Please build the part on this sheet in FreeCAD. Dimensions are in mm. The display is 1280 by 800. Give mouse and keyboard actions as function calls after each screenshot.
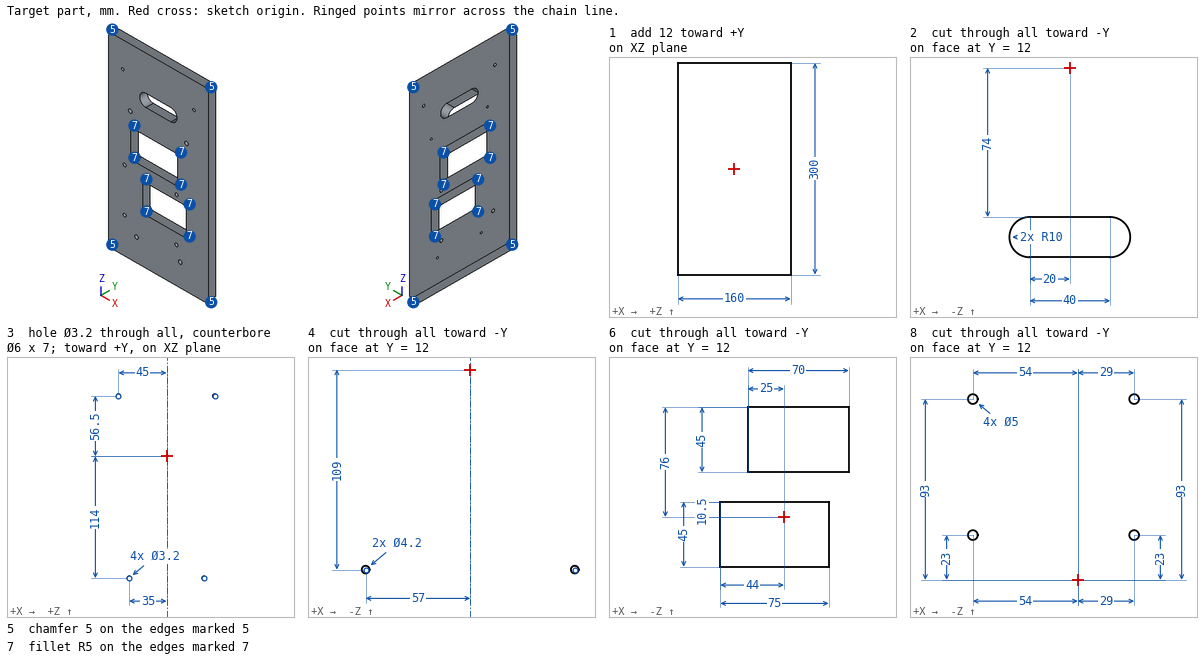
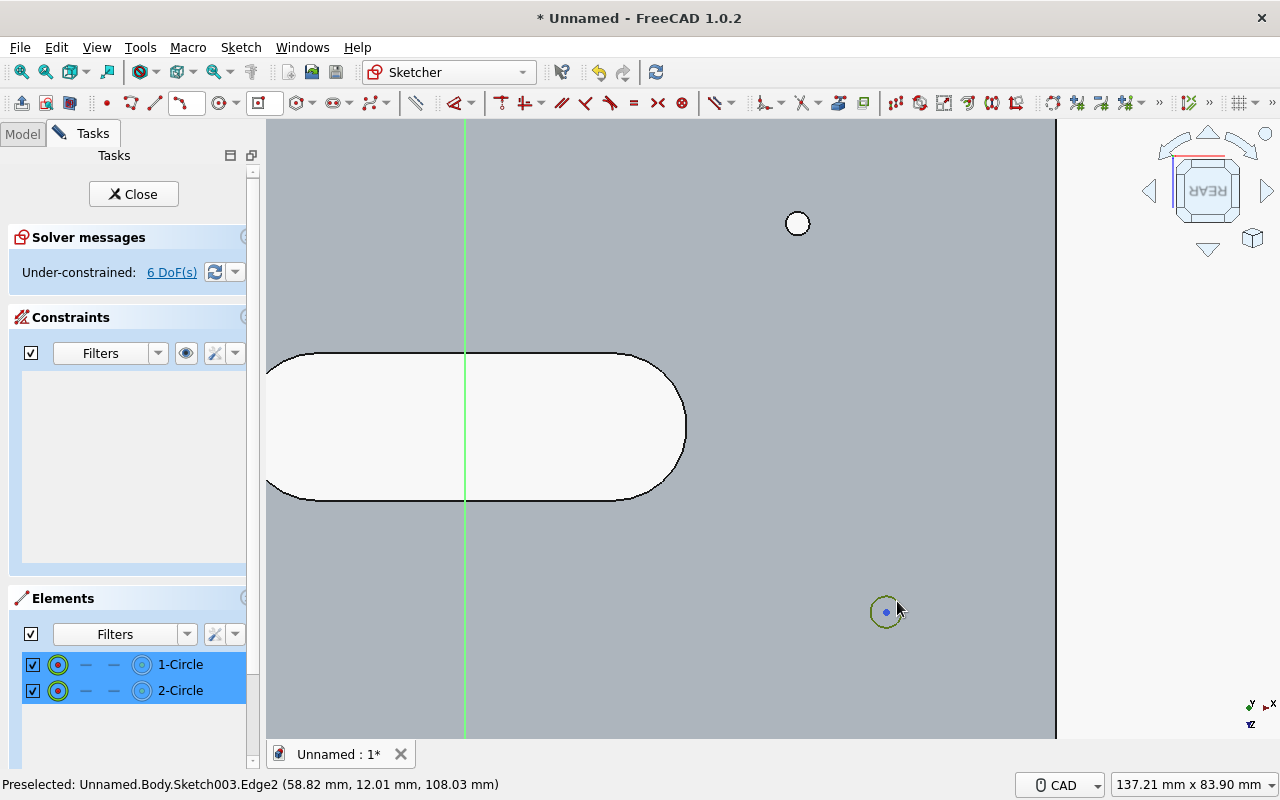
click(634, 104)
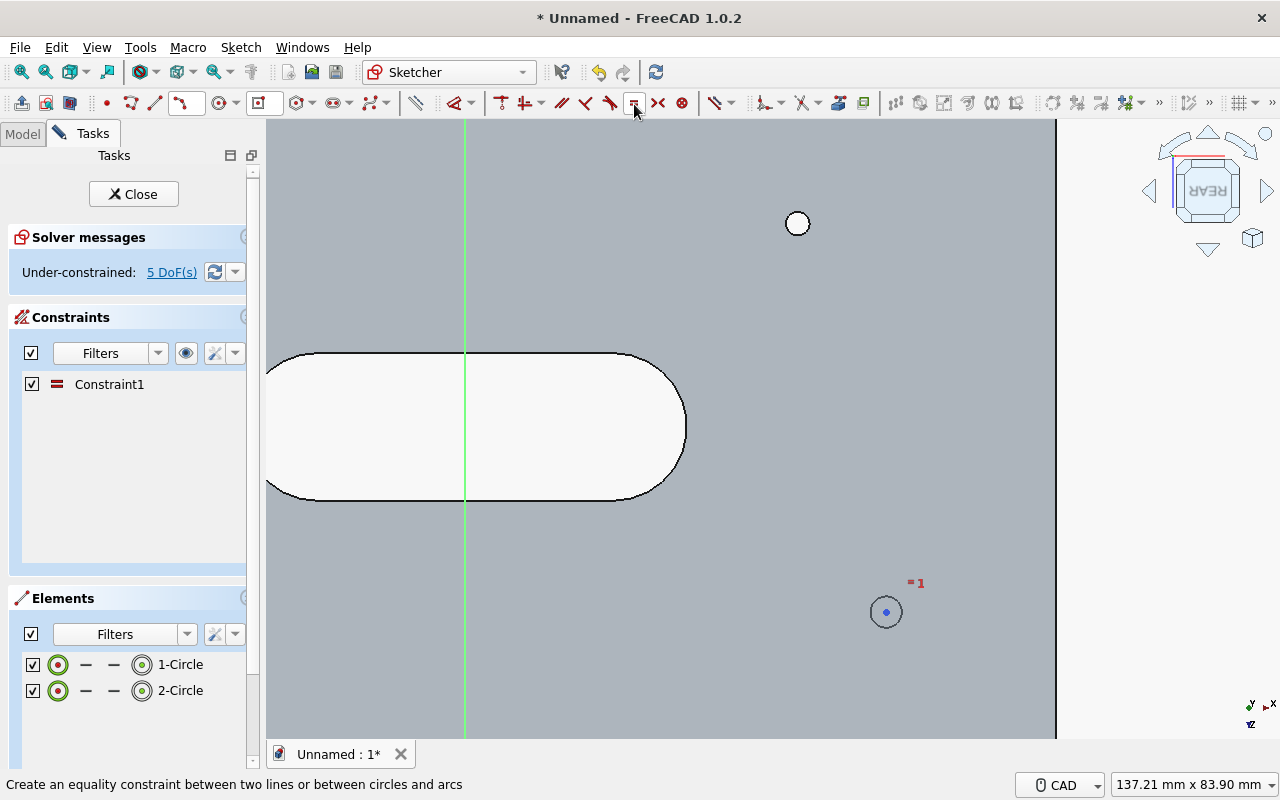
scroll(900, 602, down, 4)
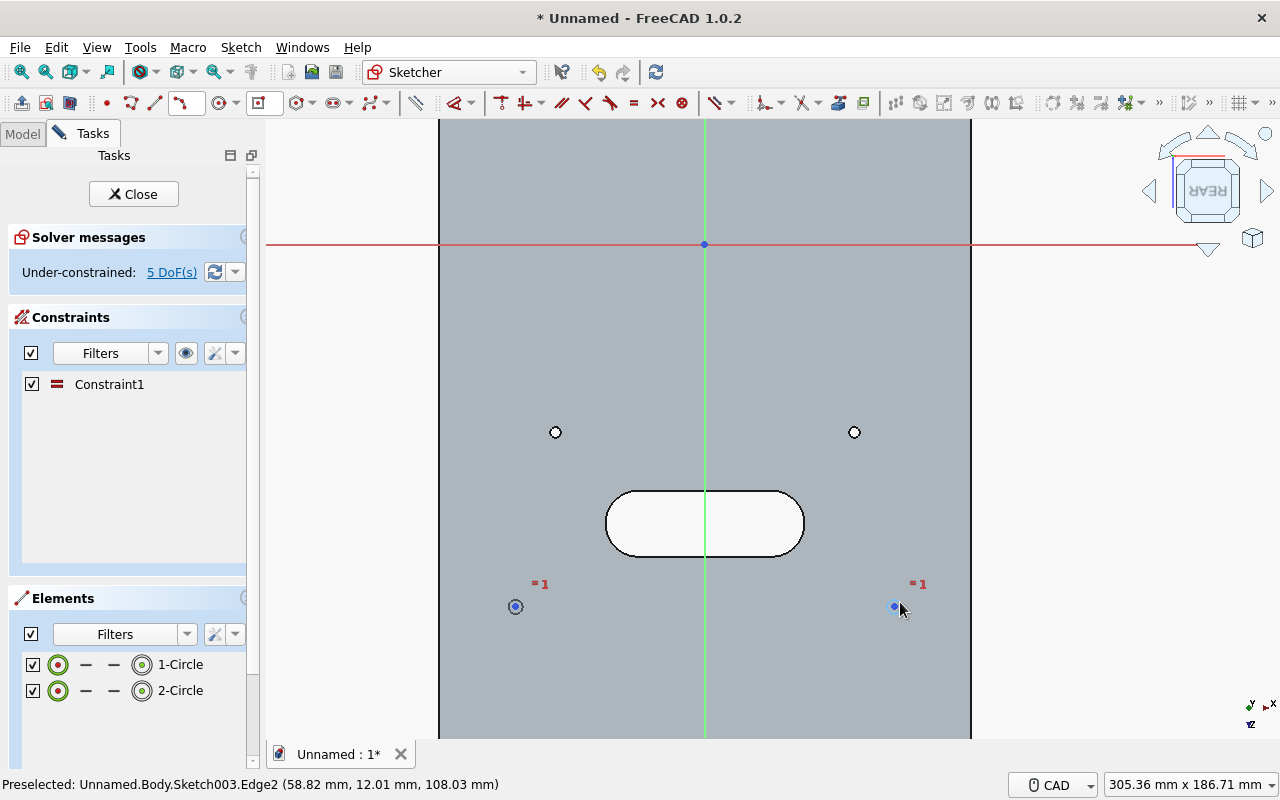
click(516, 607)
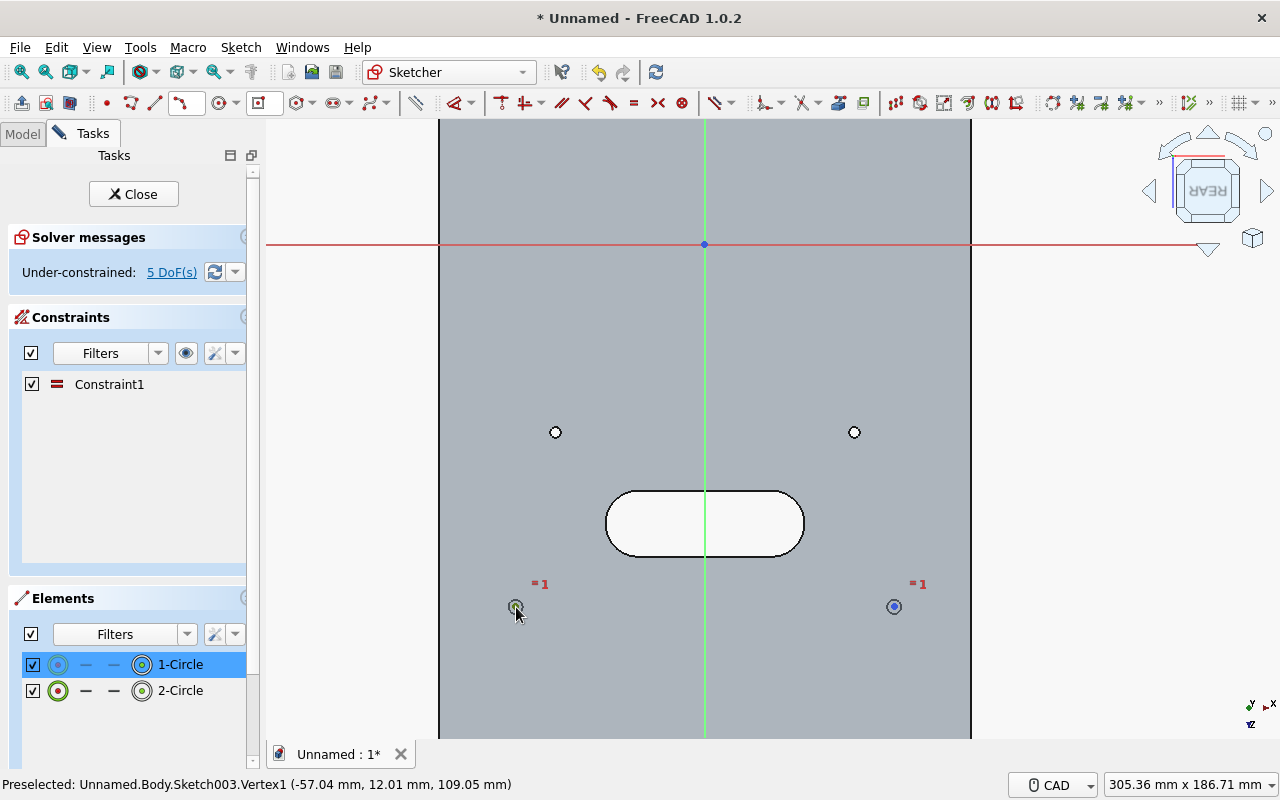
click(894, 607)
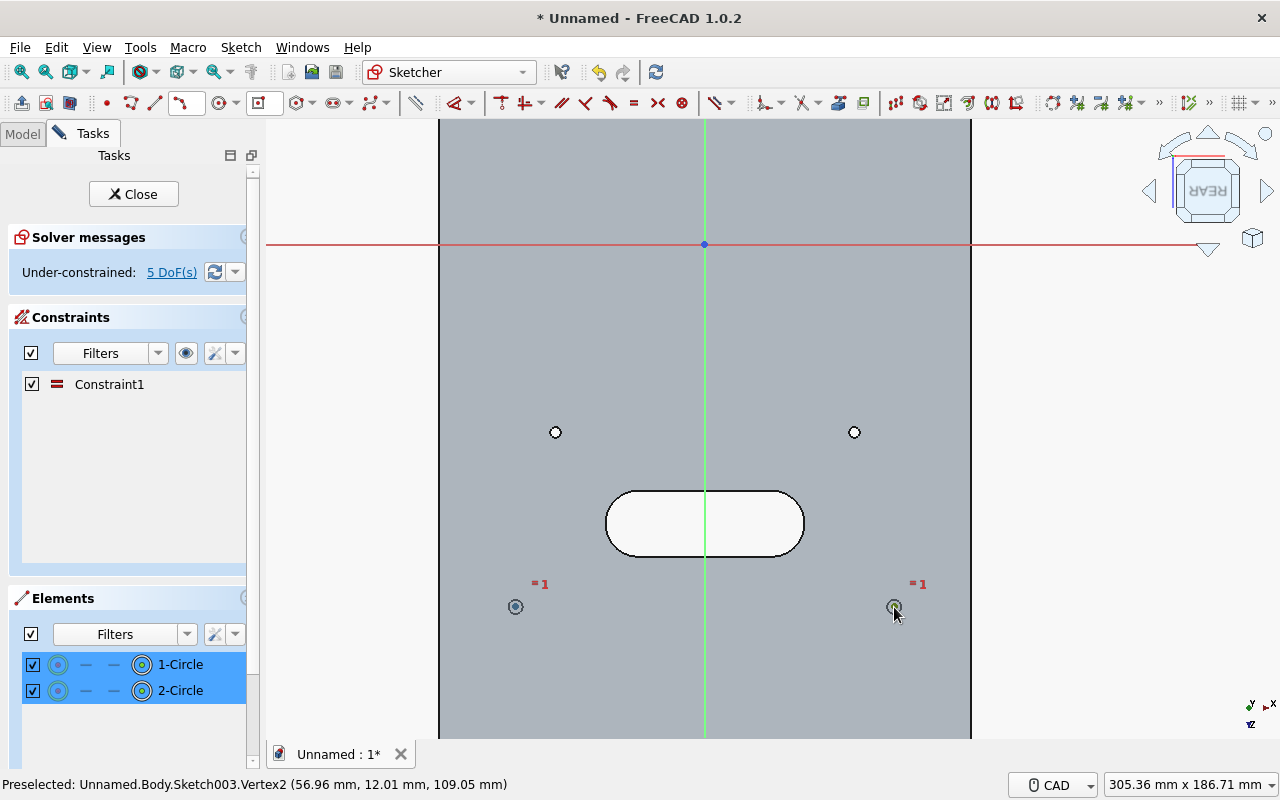
click(705, 671)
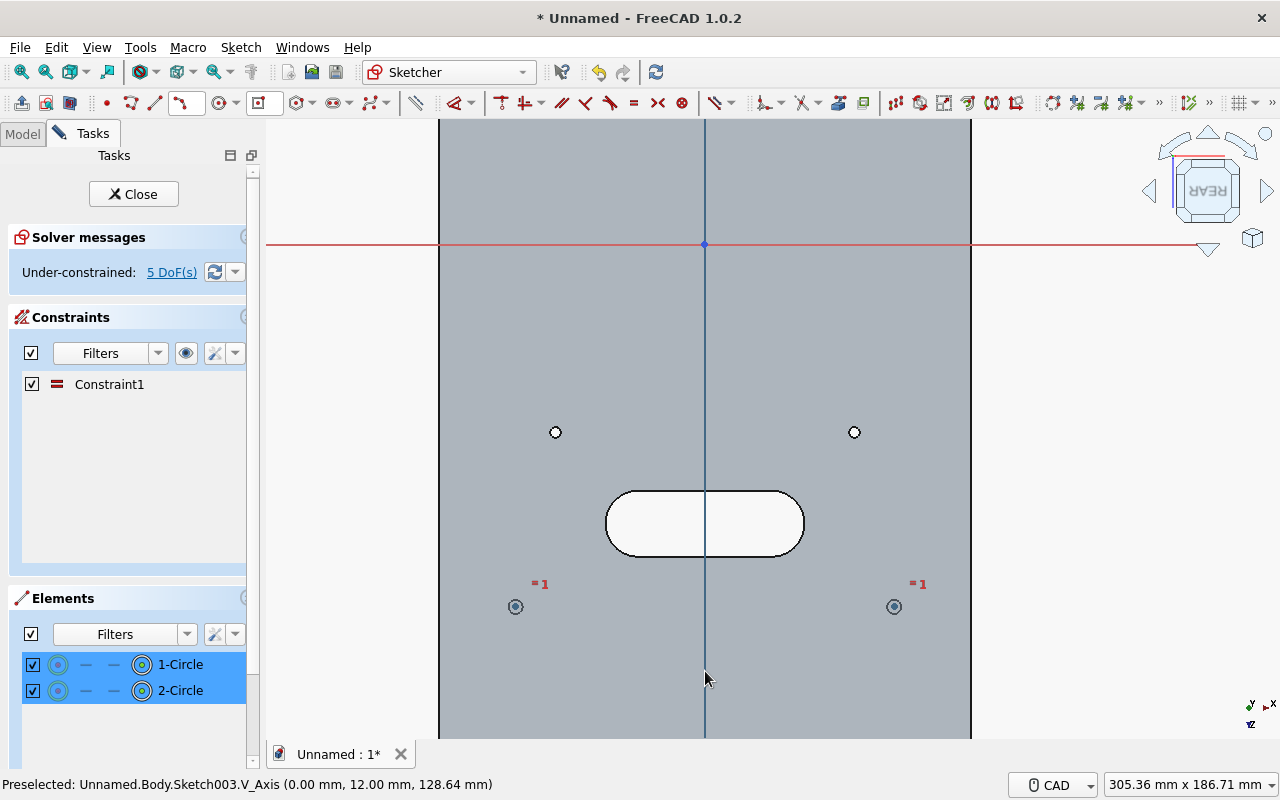
click(658, 104)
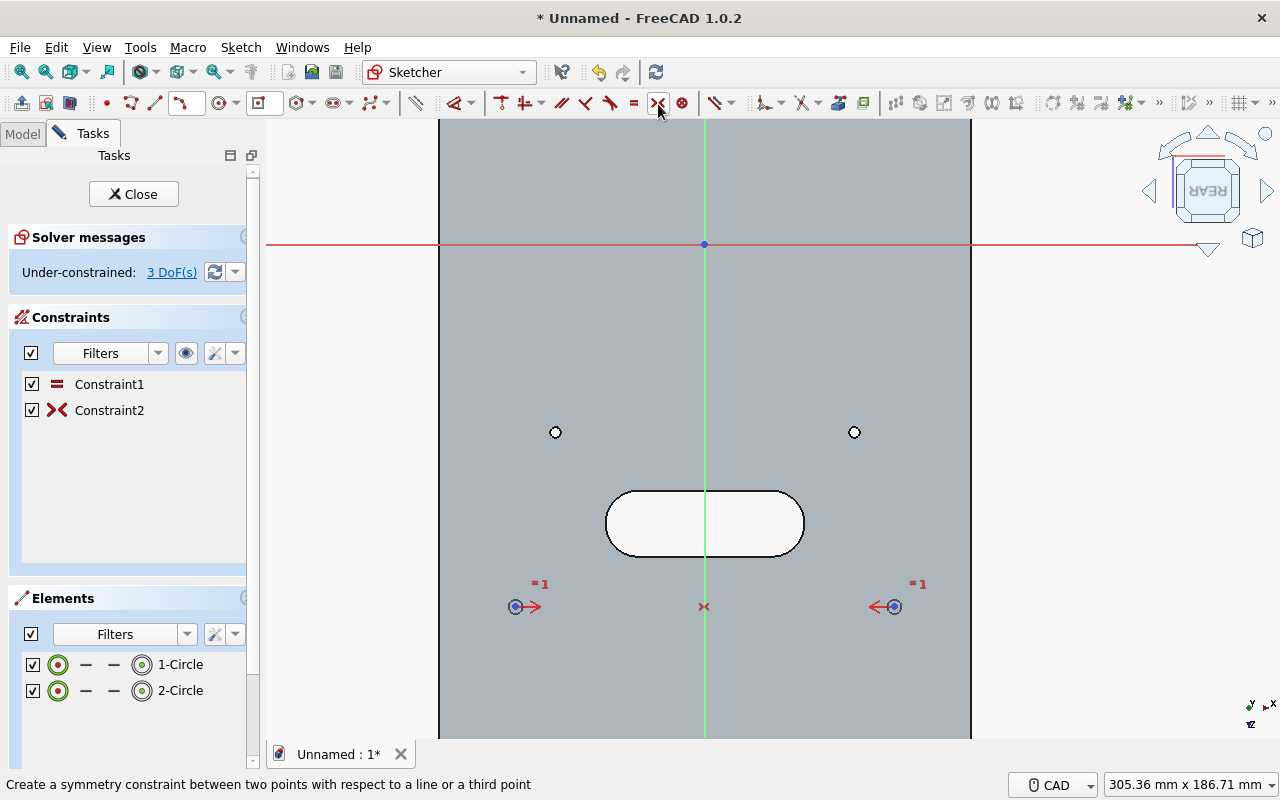
click(454, 104)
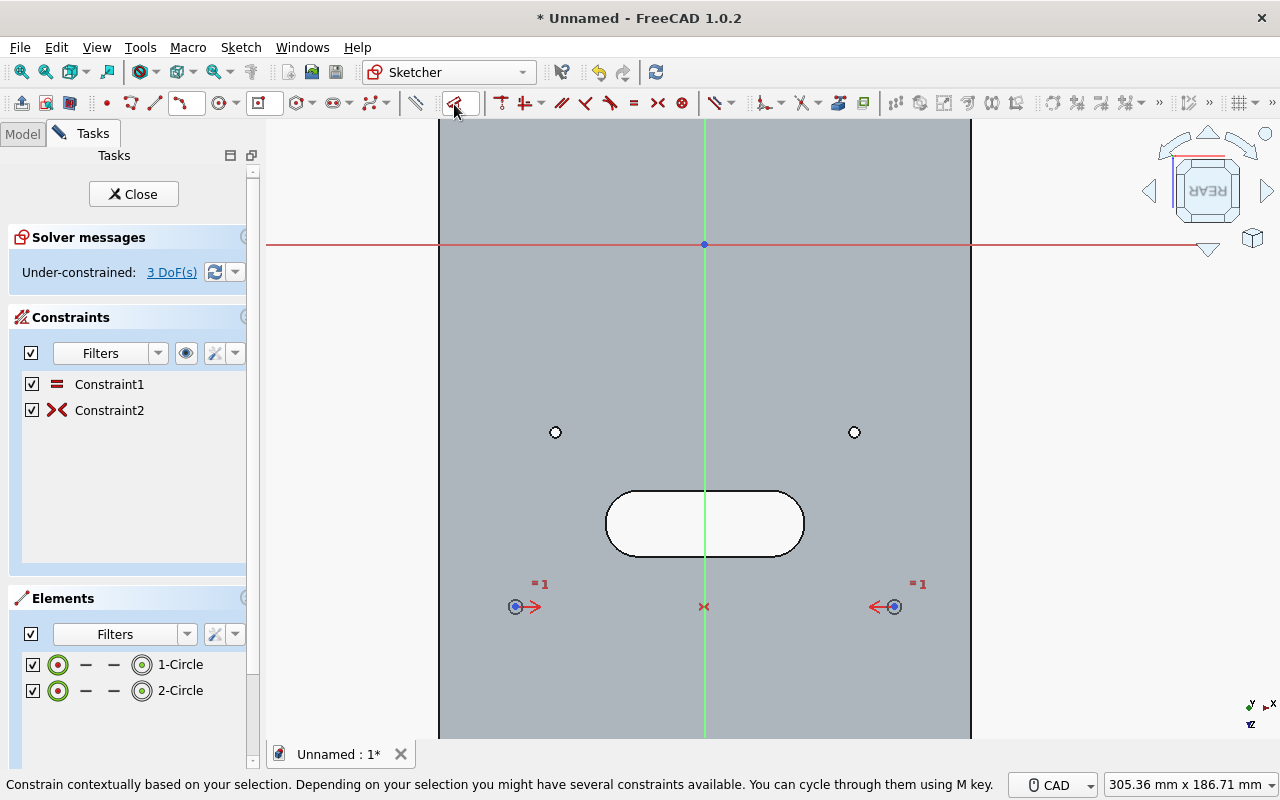
scroll(516, 600, up, 6)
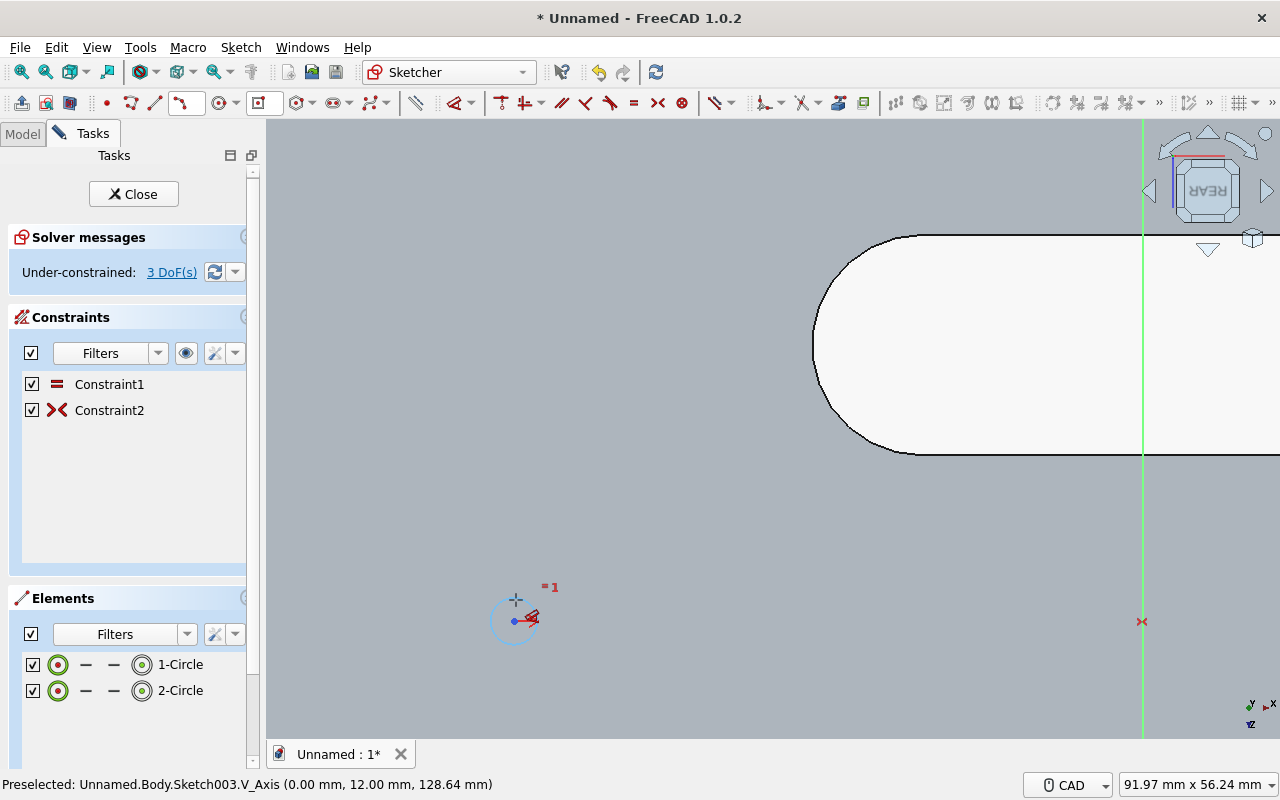
click(515, 598)
click(516, 566)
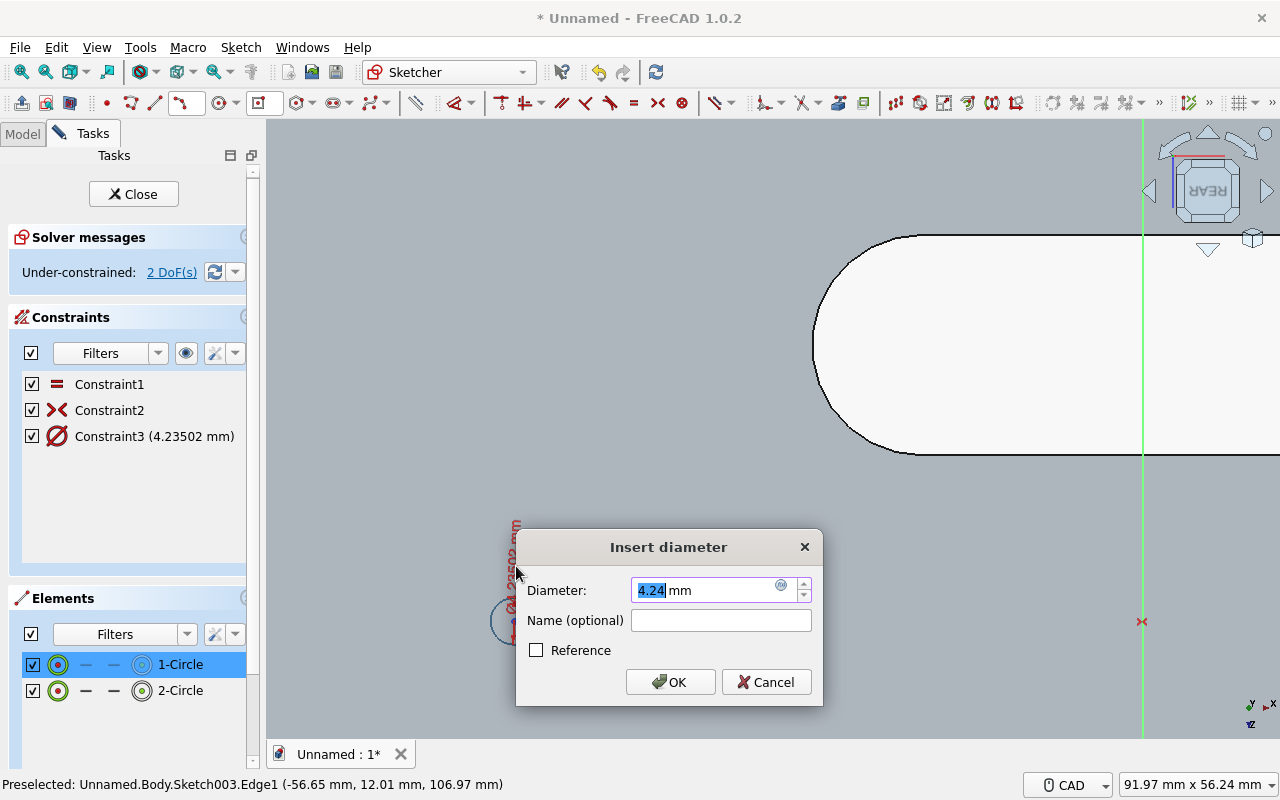
text(4.2)
key(Return)